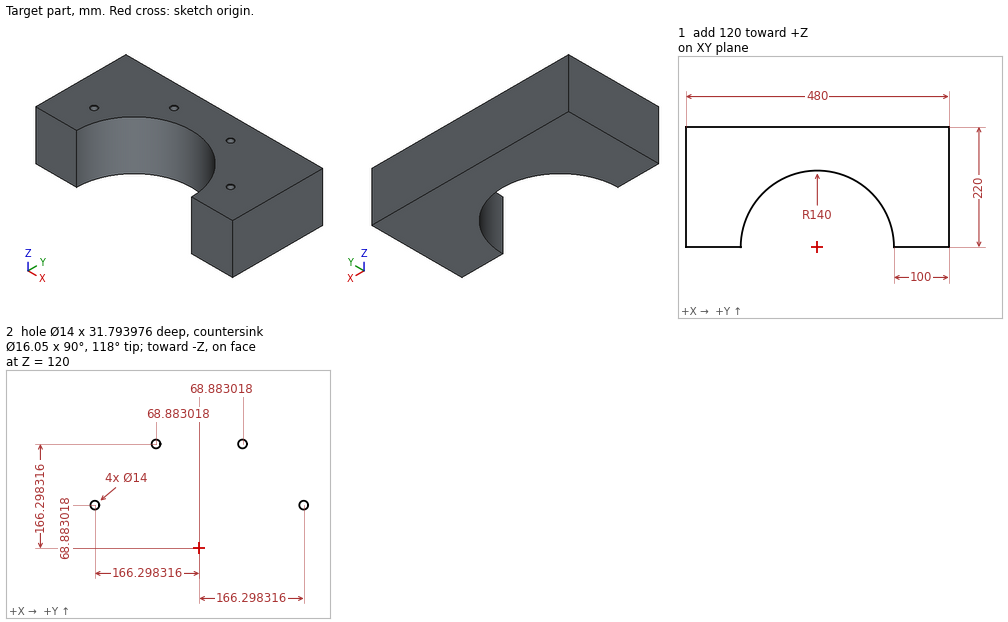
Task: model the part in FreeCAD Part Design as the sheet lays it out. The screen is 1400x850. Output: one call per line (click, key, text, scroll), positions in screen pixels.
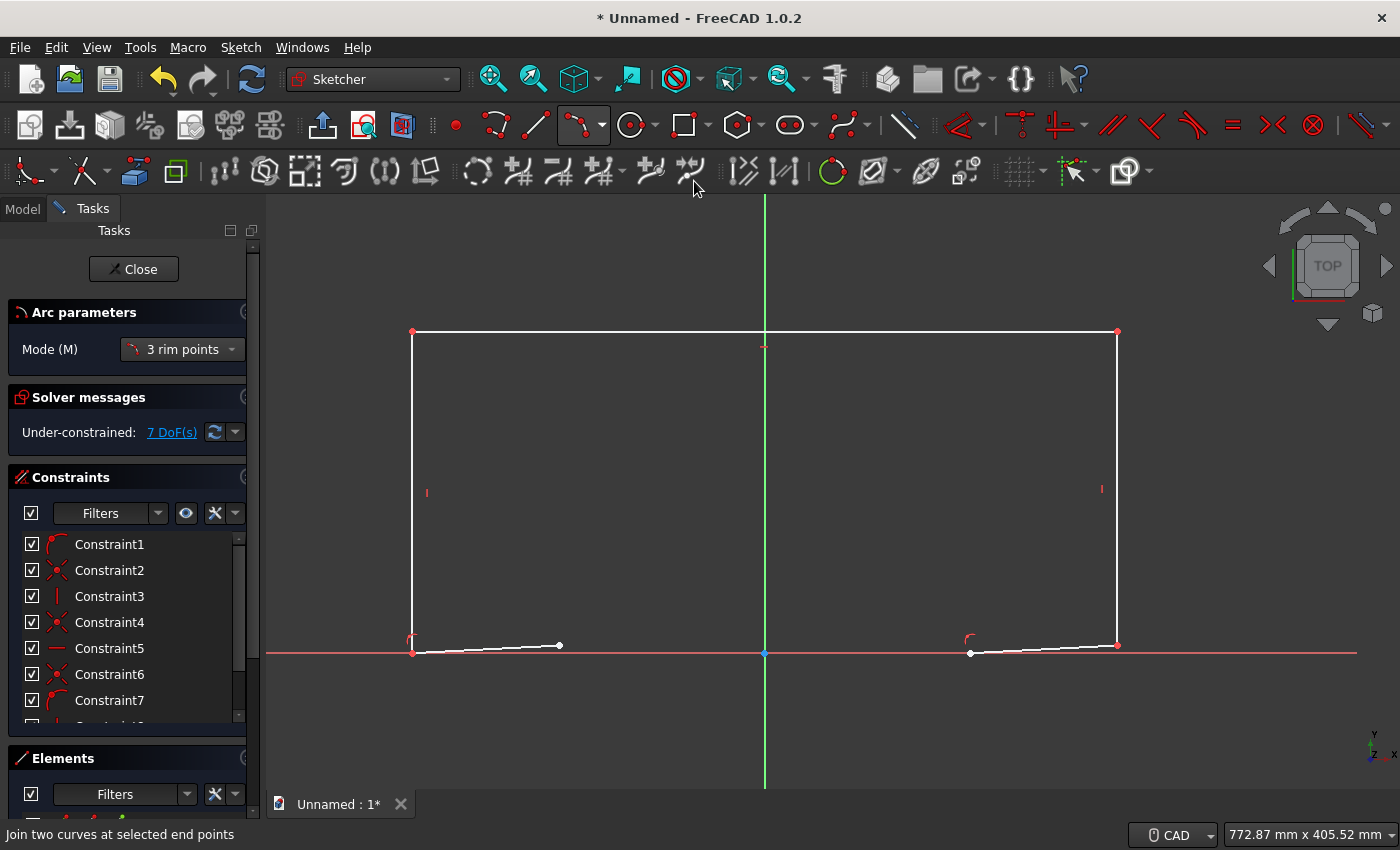
click(560, 645)
click(971, 653)
click(828, 458)
key(Escape)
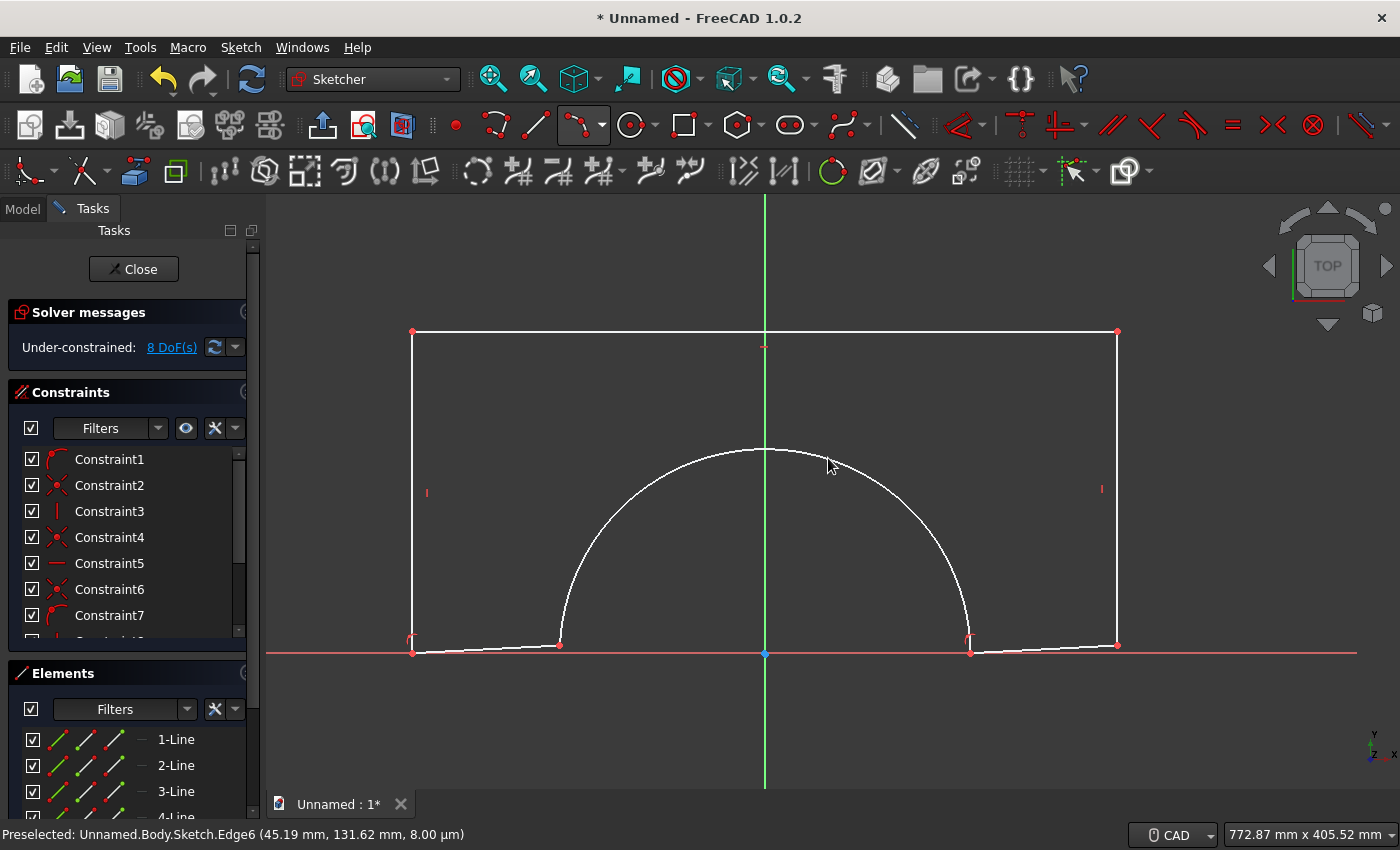
click(1014, 651)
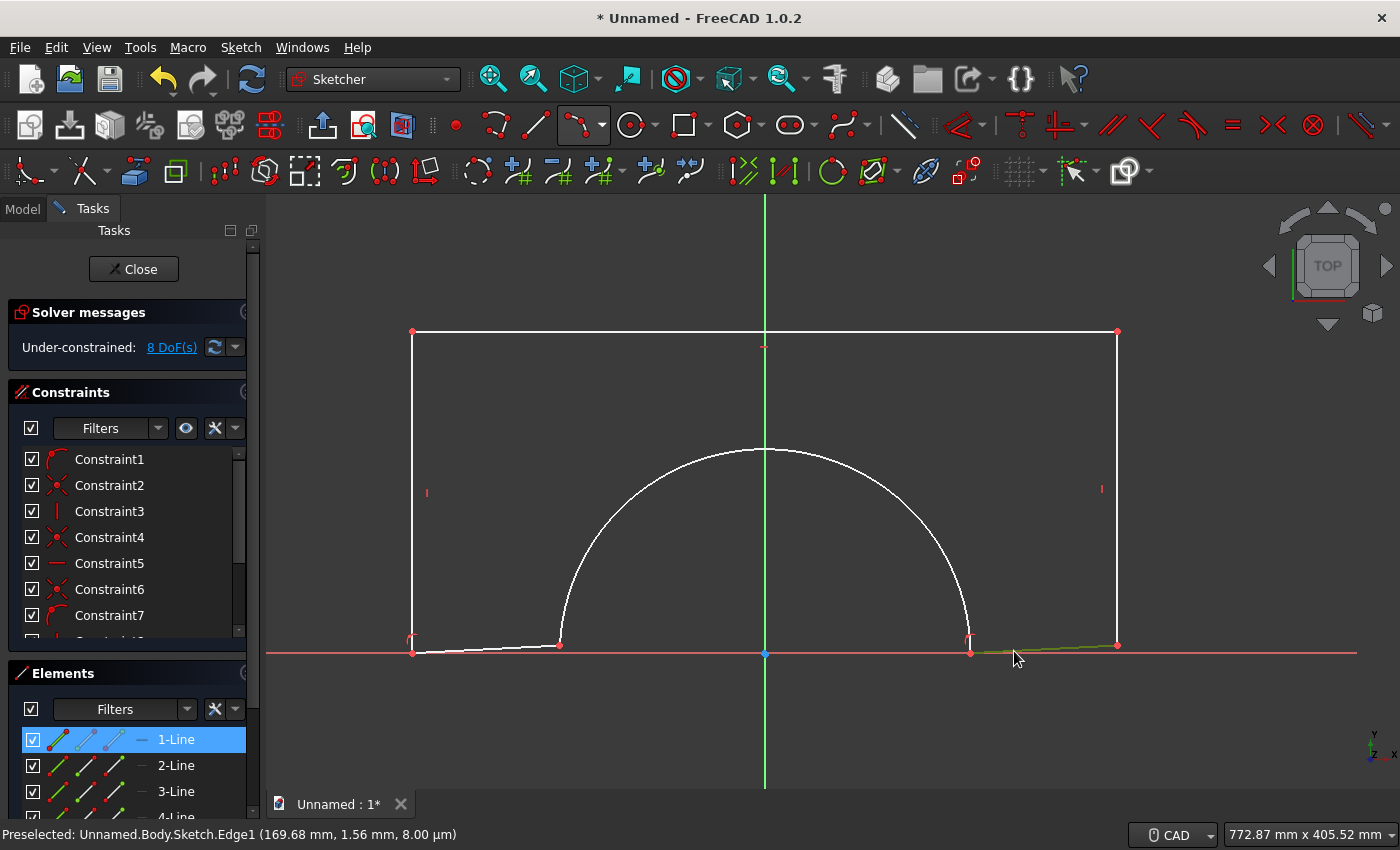
key(h)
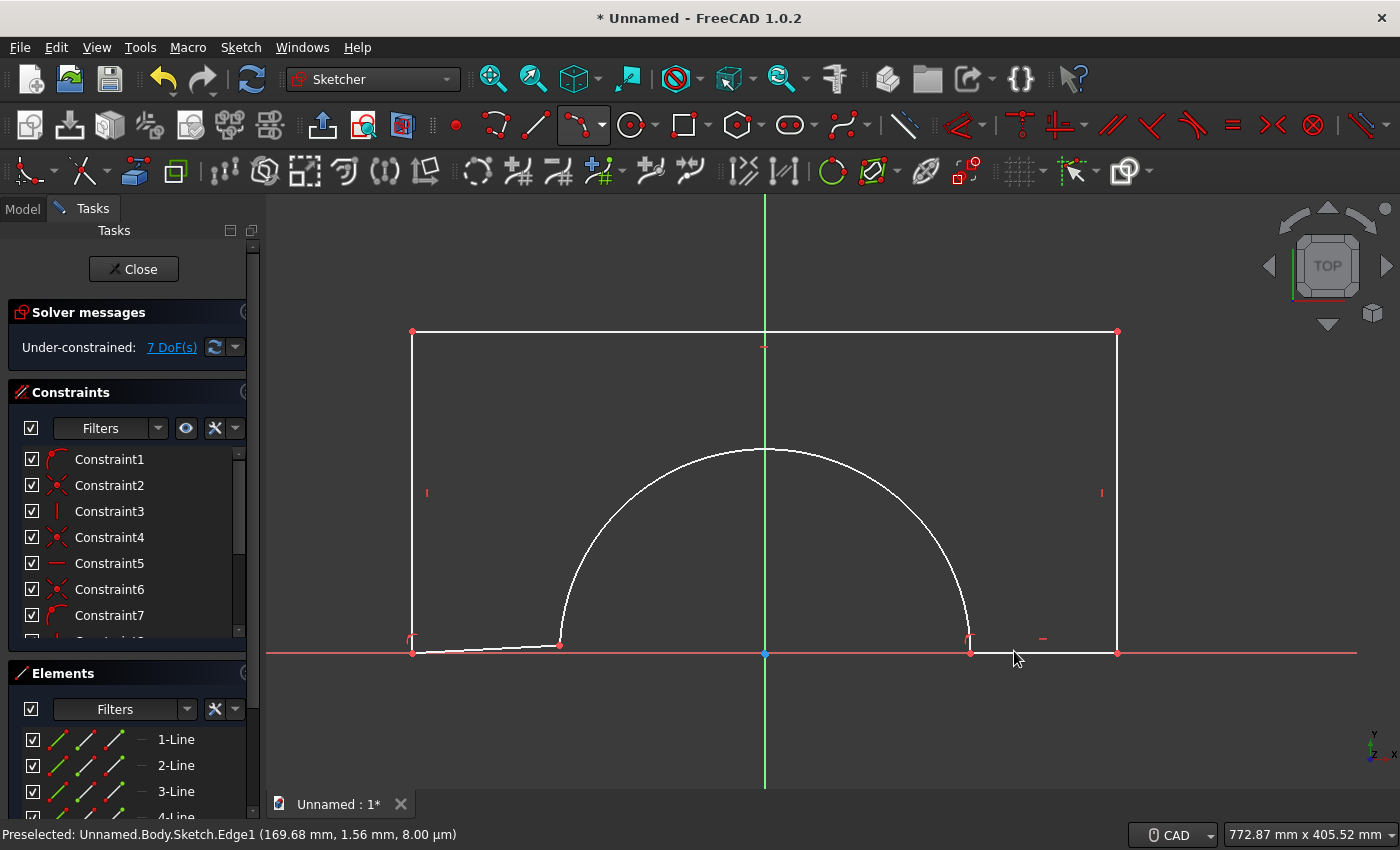
click(457, 651)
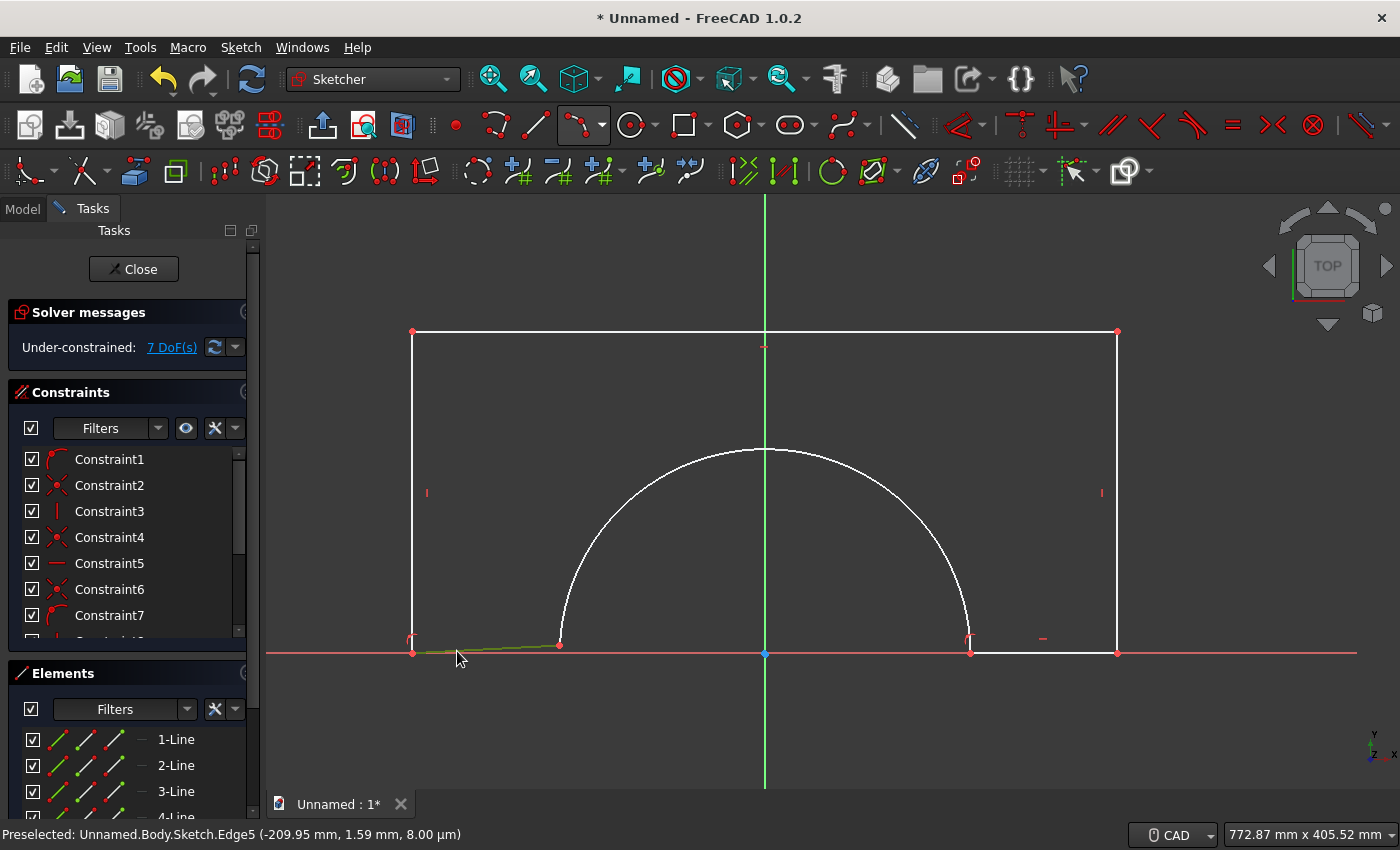
click(1086, 126)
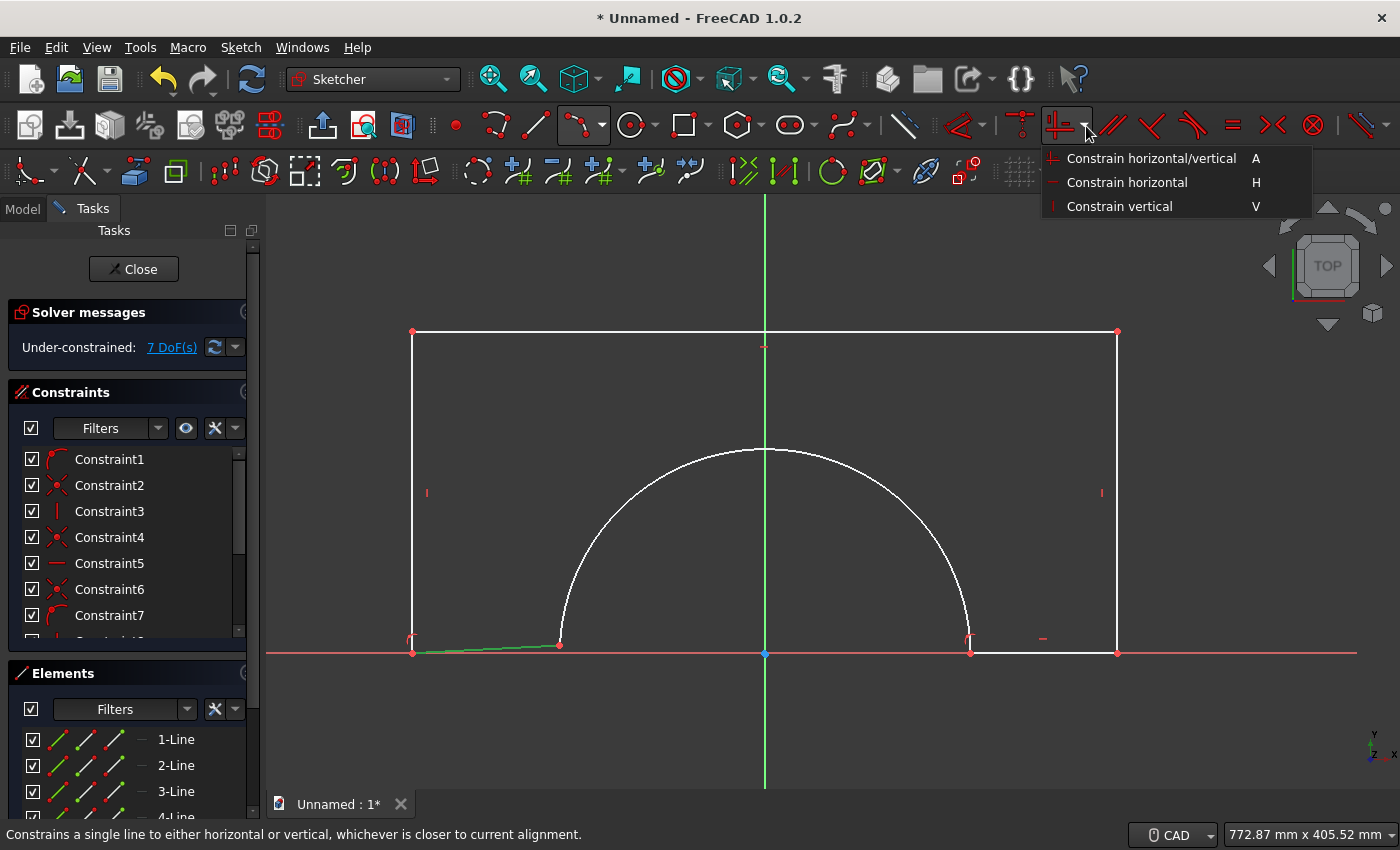
click(1177, 182)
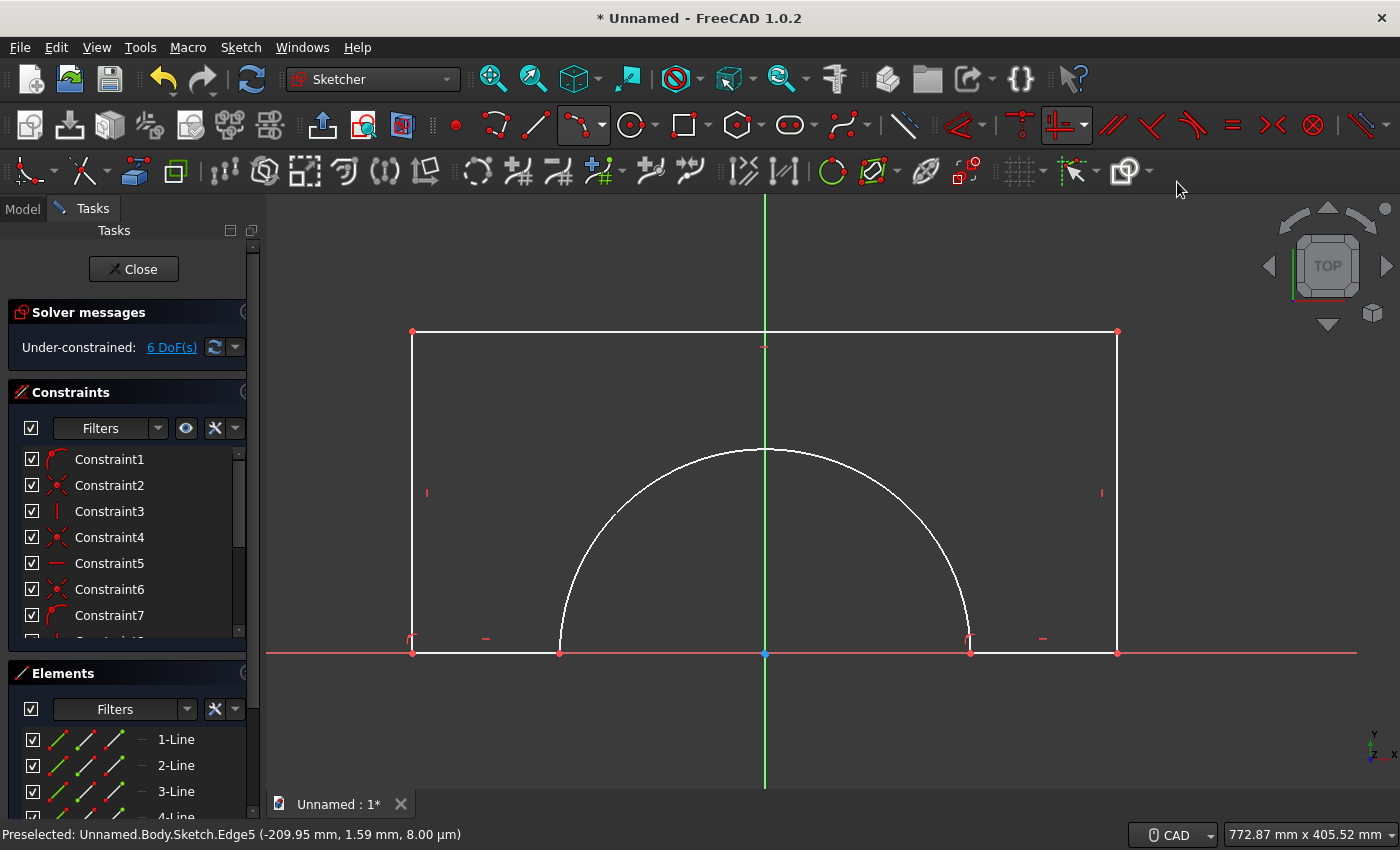
drag(755, 643, 775, 665)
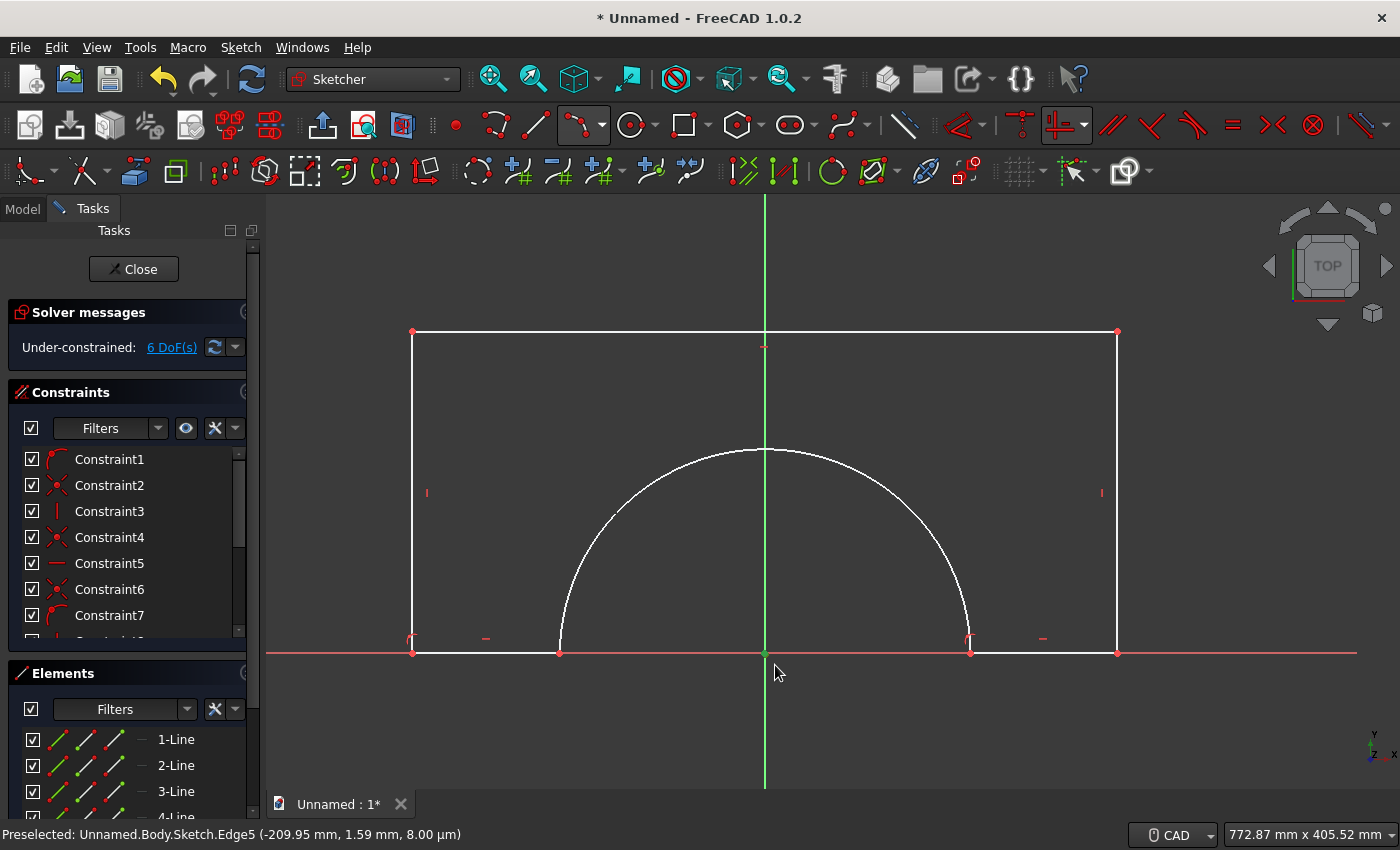
key(c)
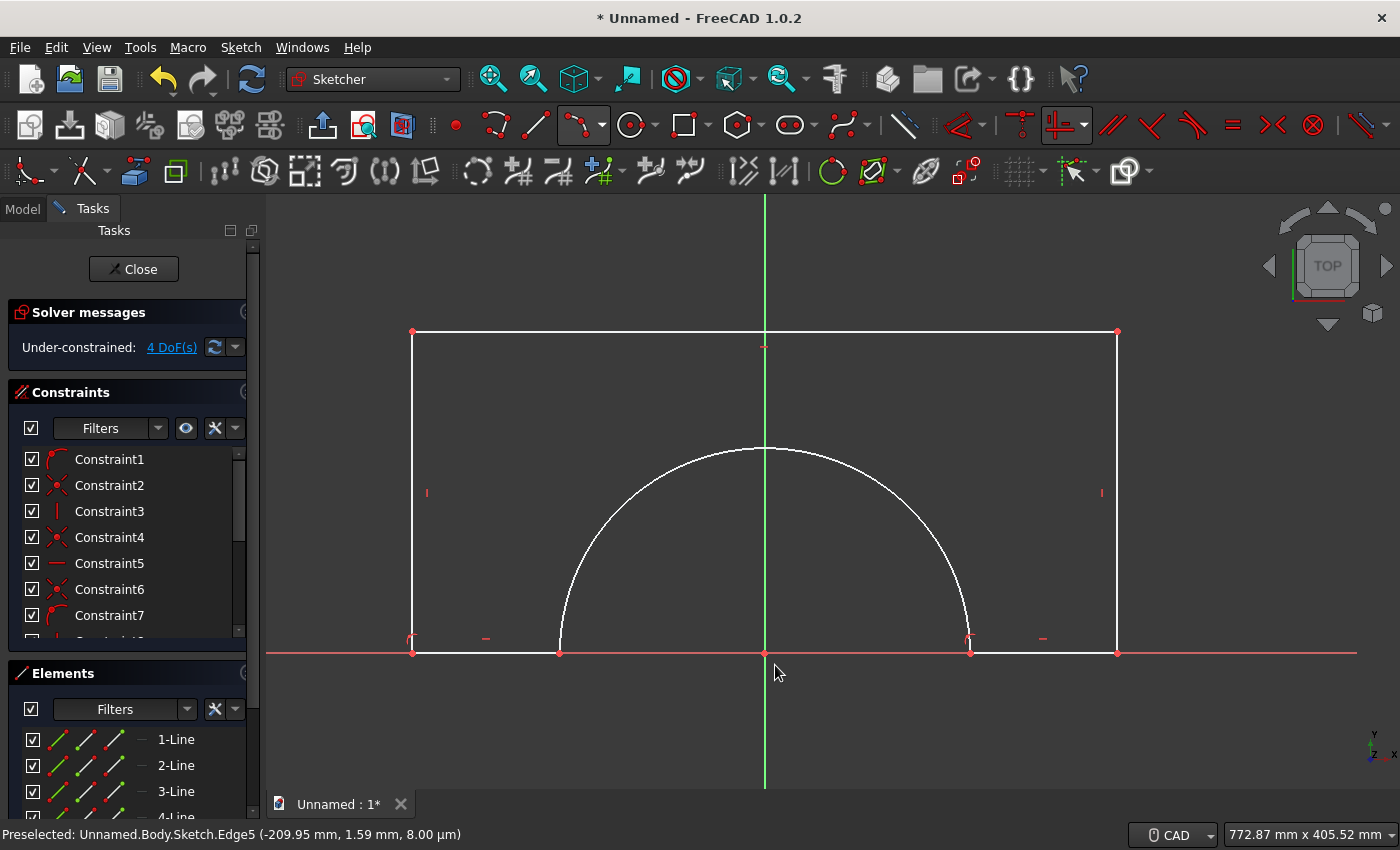
click(958, 126)